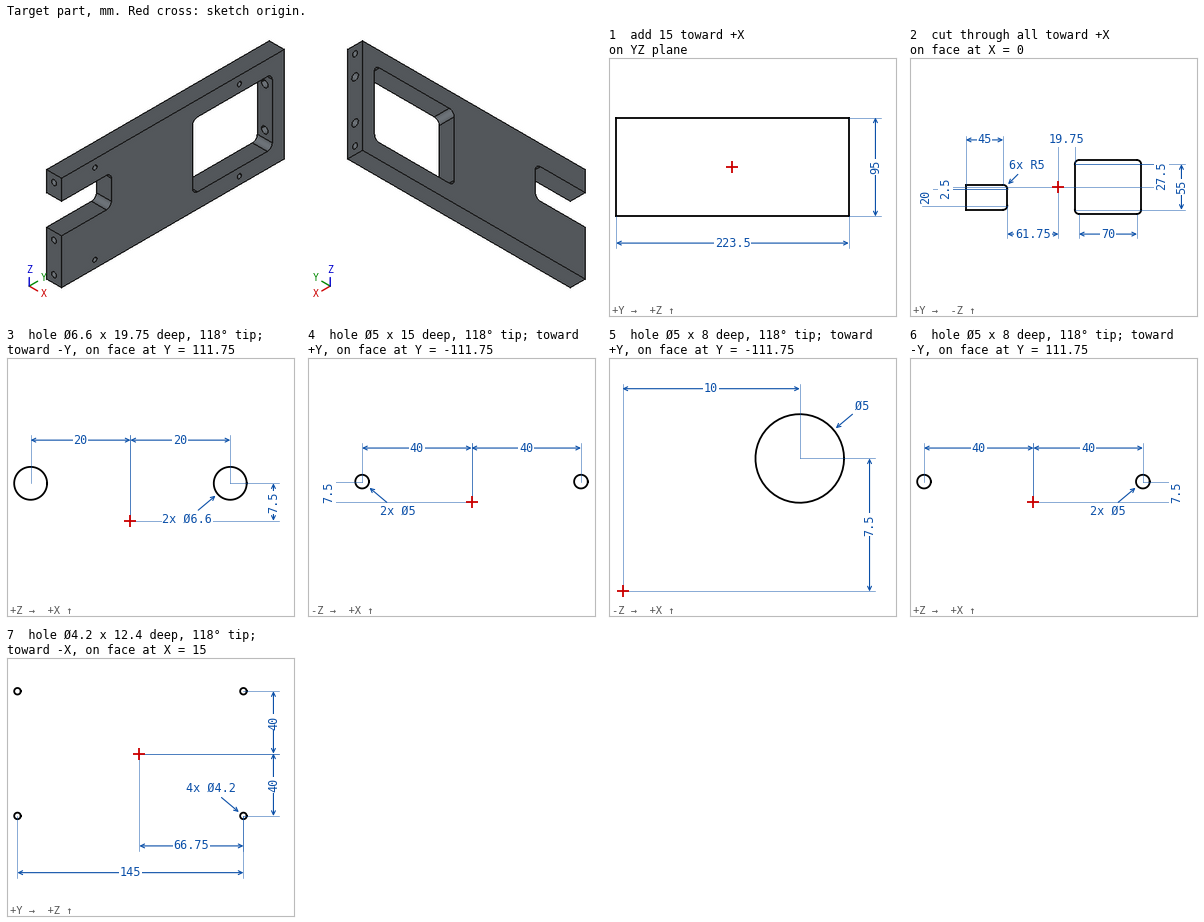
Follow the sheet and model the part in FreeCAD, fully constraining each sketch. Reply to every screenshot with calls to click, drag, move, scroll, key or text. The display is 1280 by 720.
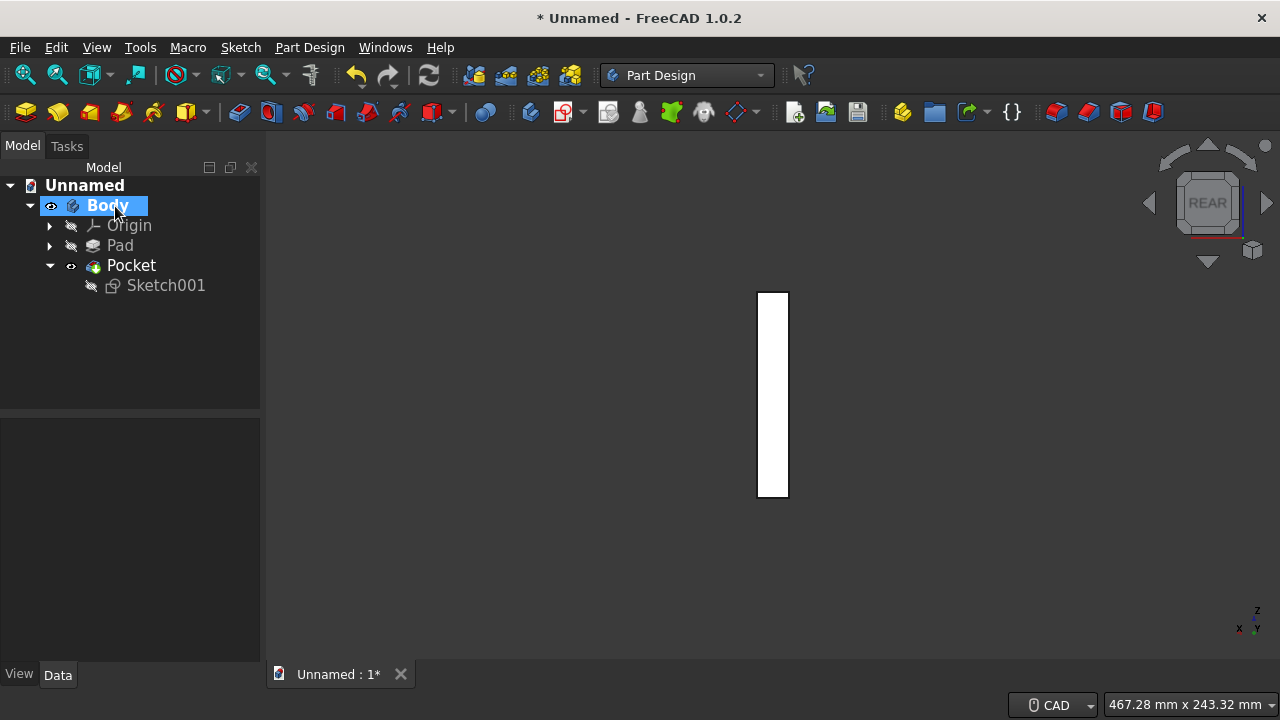
click(26, 76)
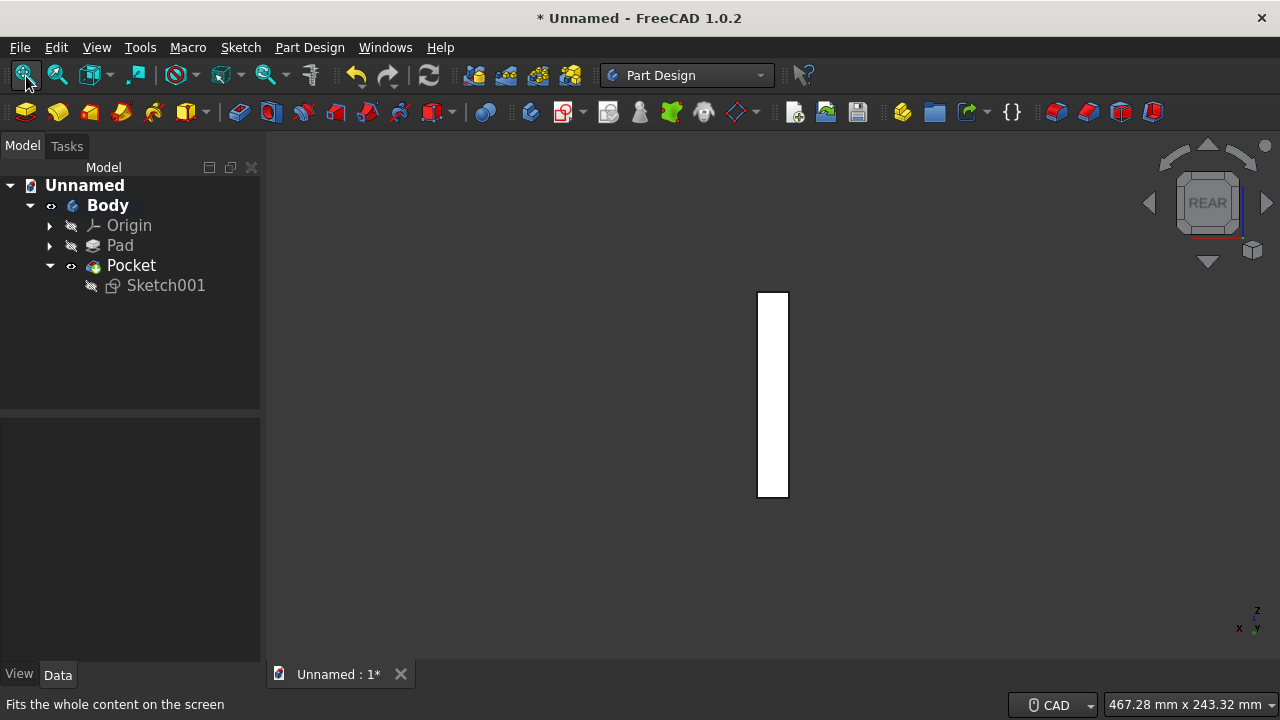
click(773, 394)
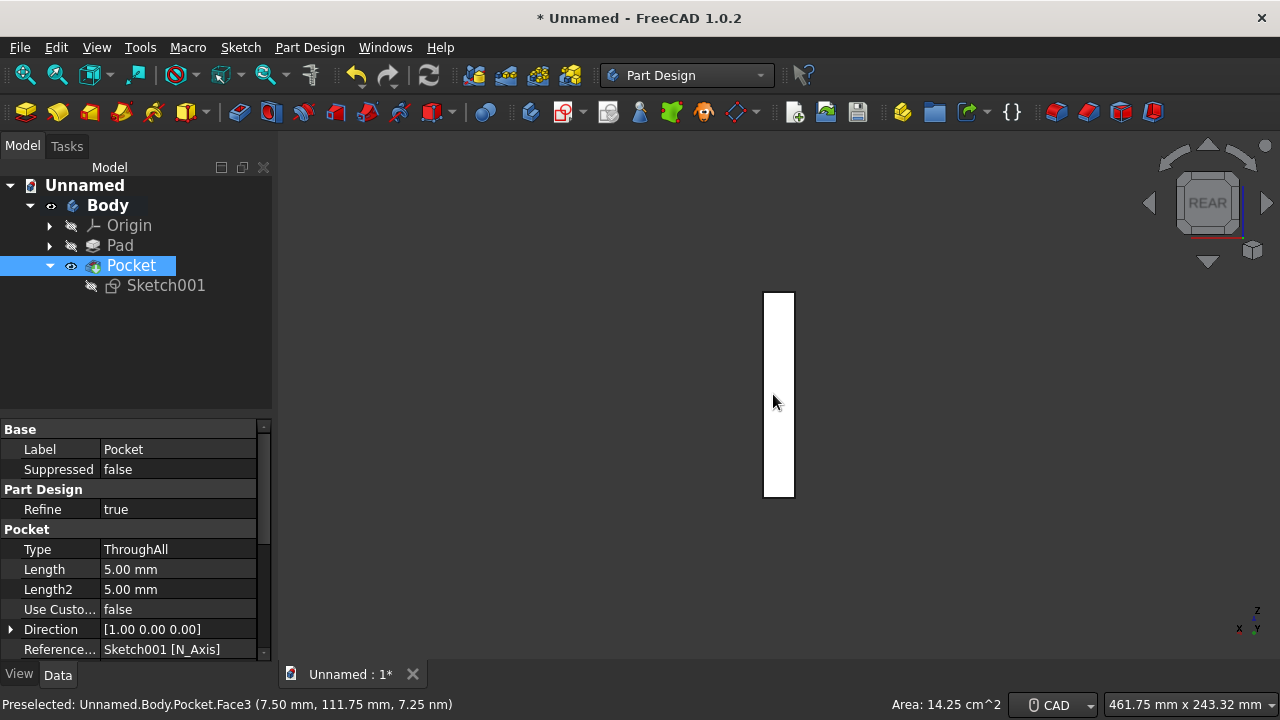
click(564, 112)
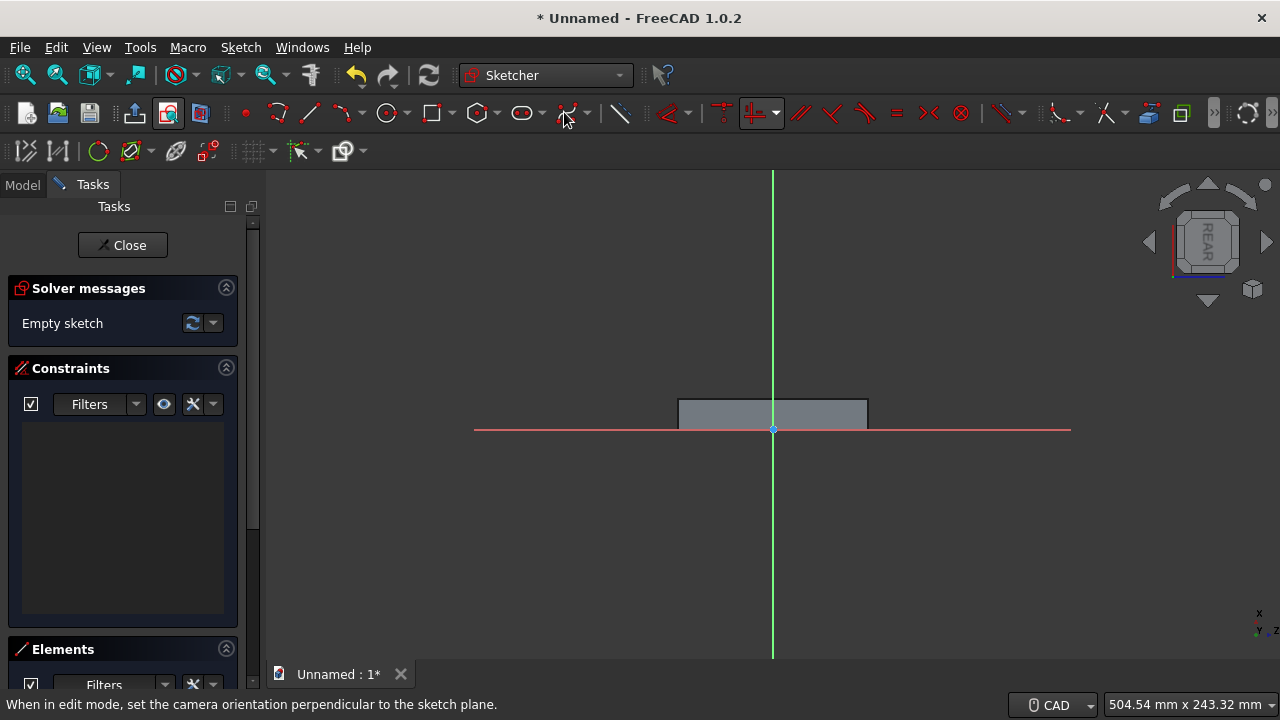
scroll(787, 420, up, 9)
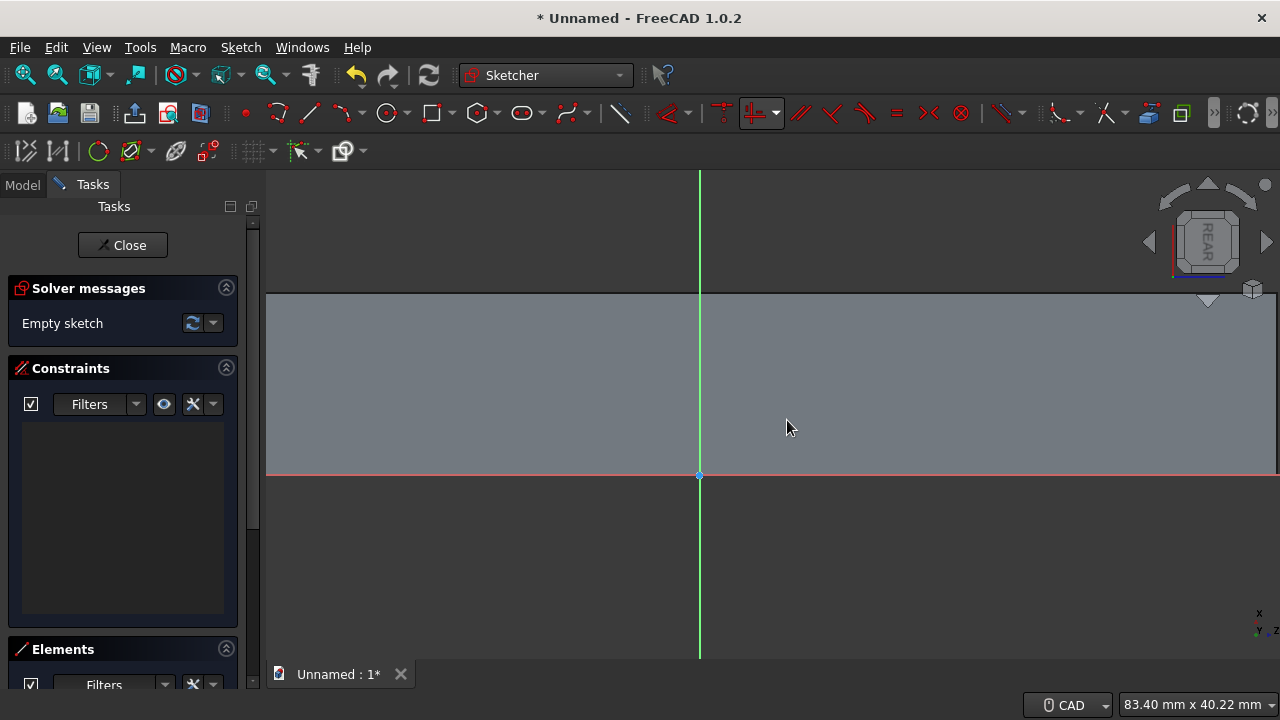
click(388, 114)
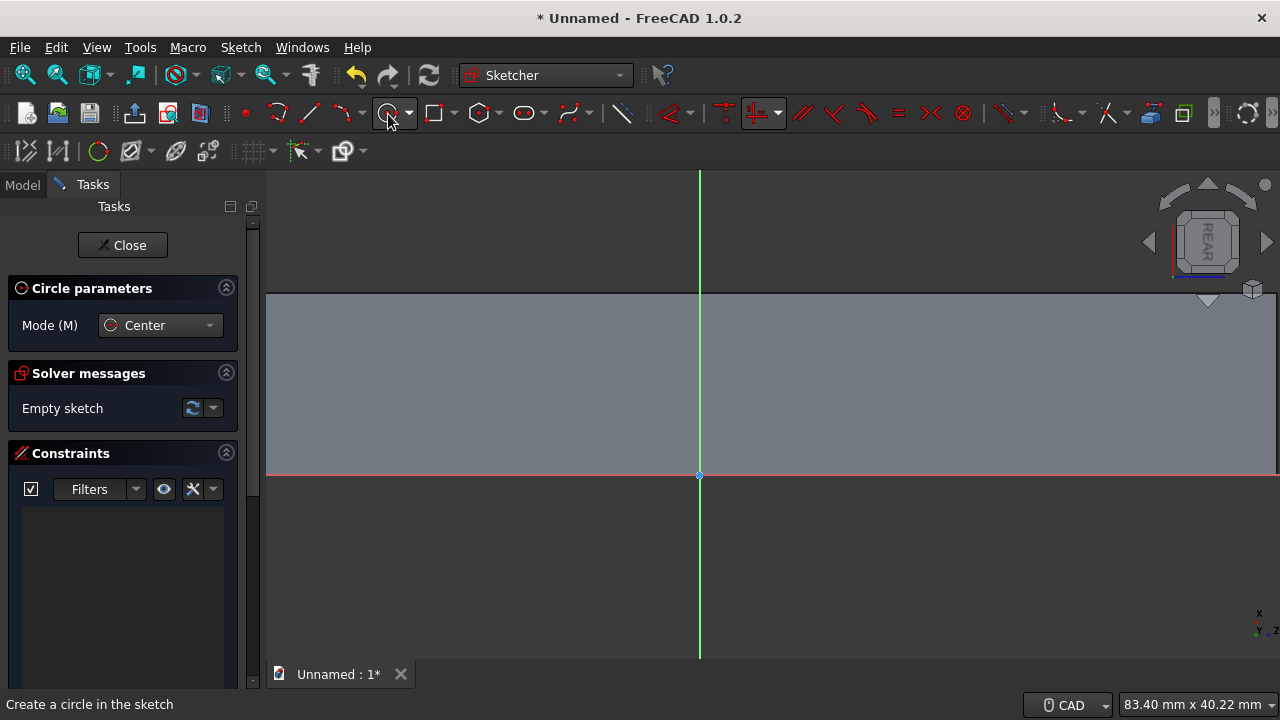
click(943, 384)
move(971, 356)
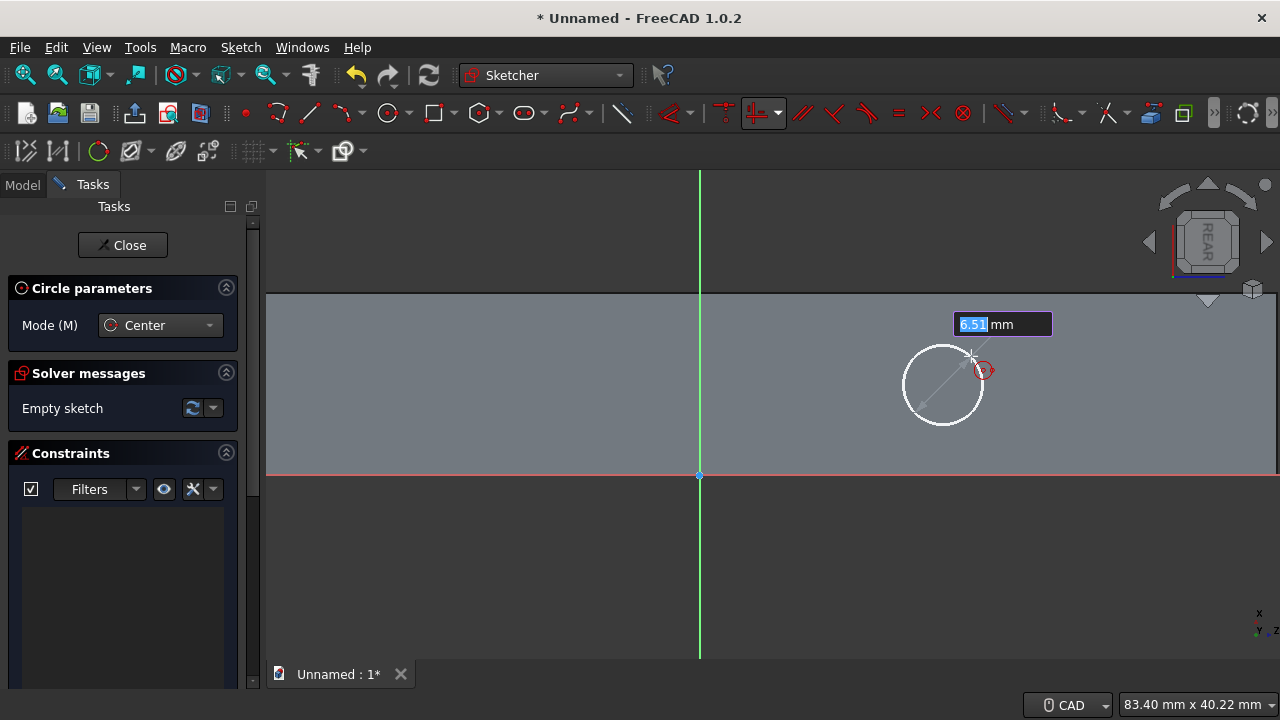
text(6.6)
key(Return)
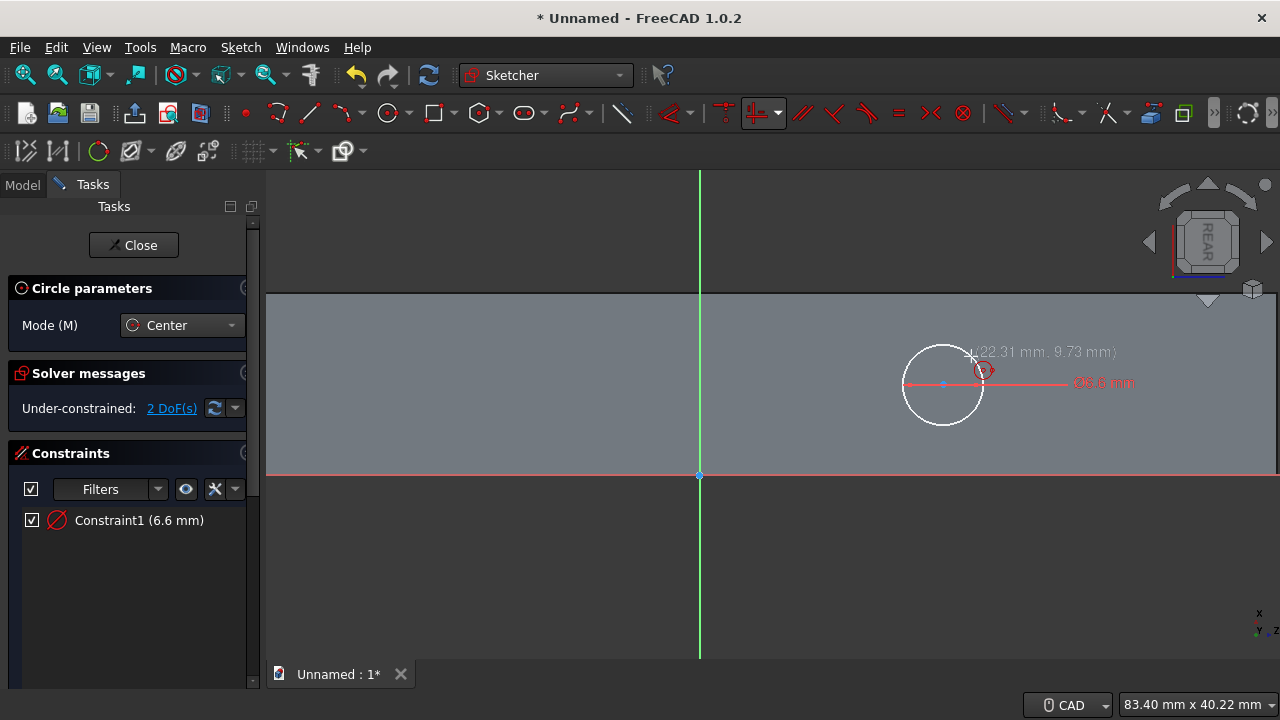
click(457, 384)
move(485, 356)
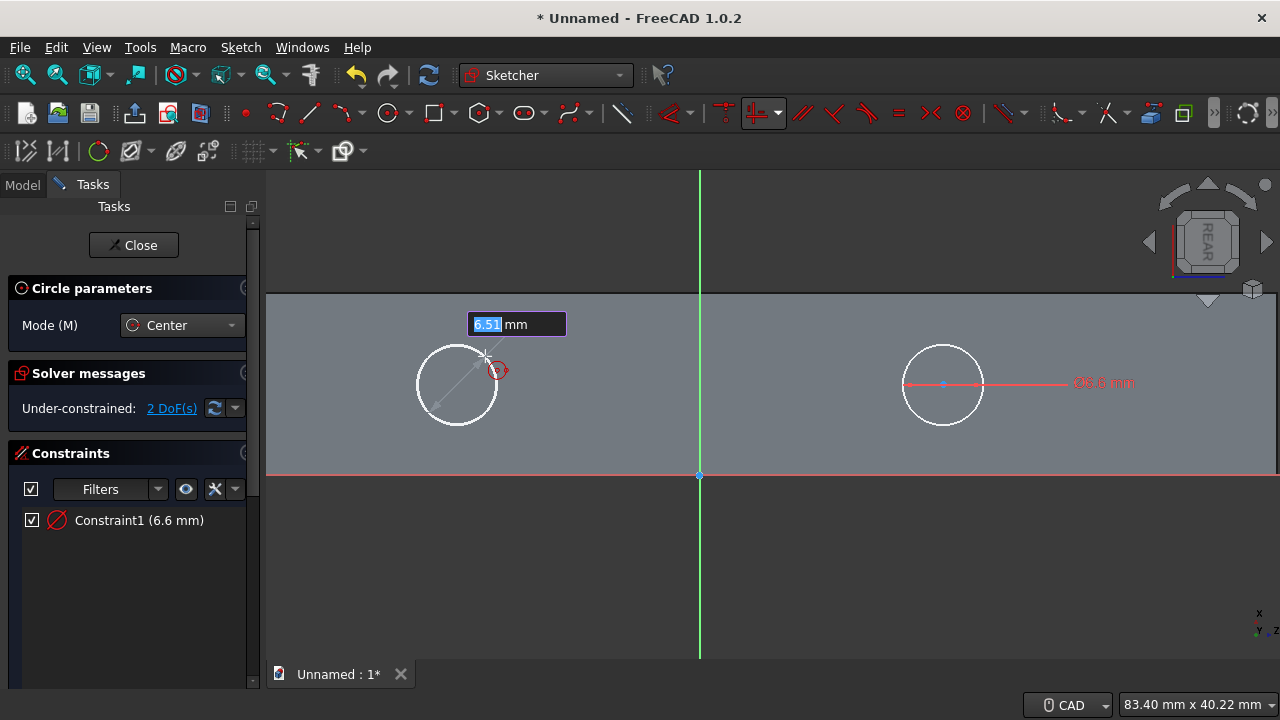
text(6.6)
key(Return)
key(Escape)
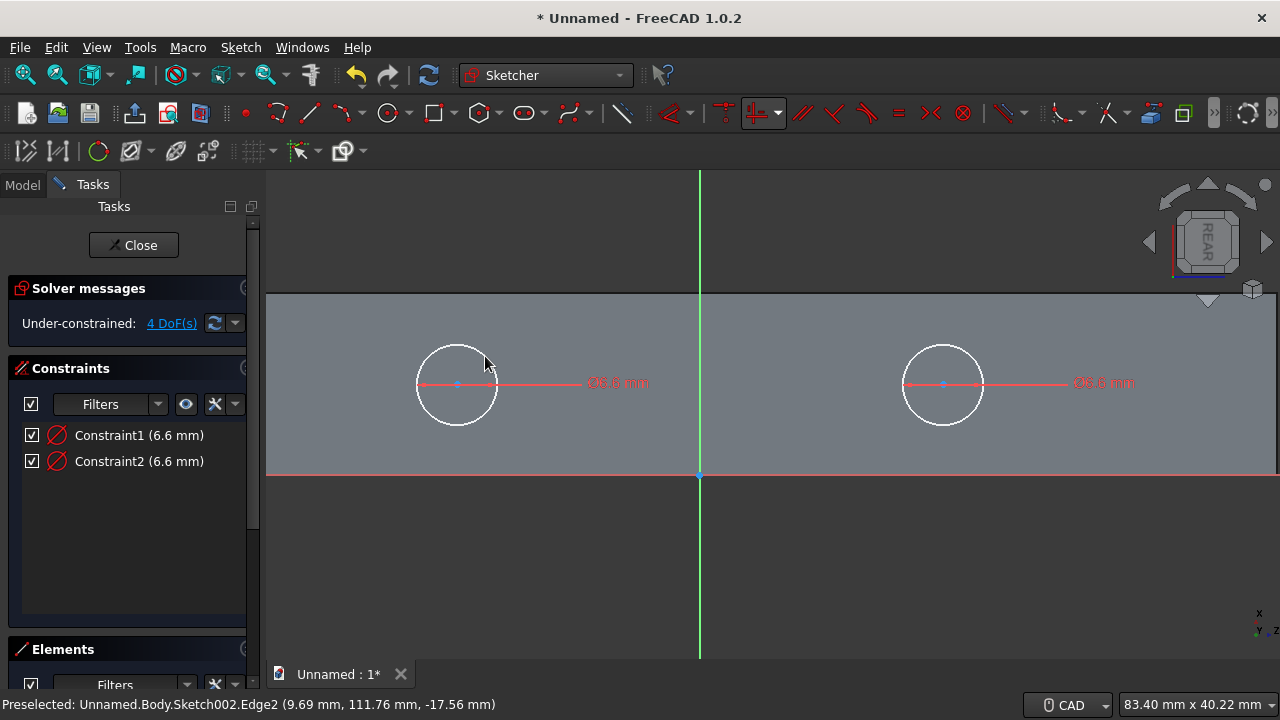
click(943, 385)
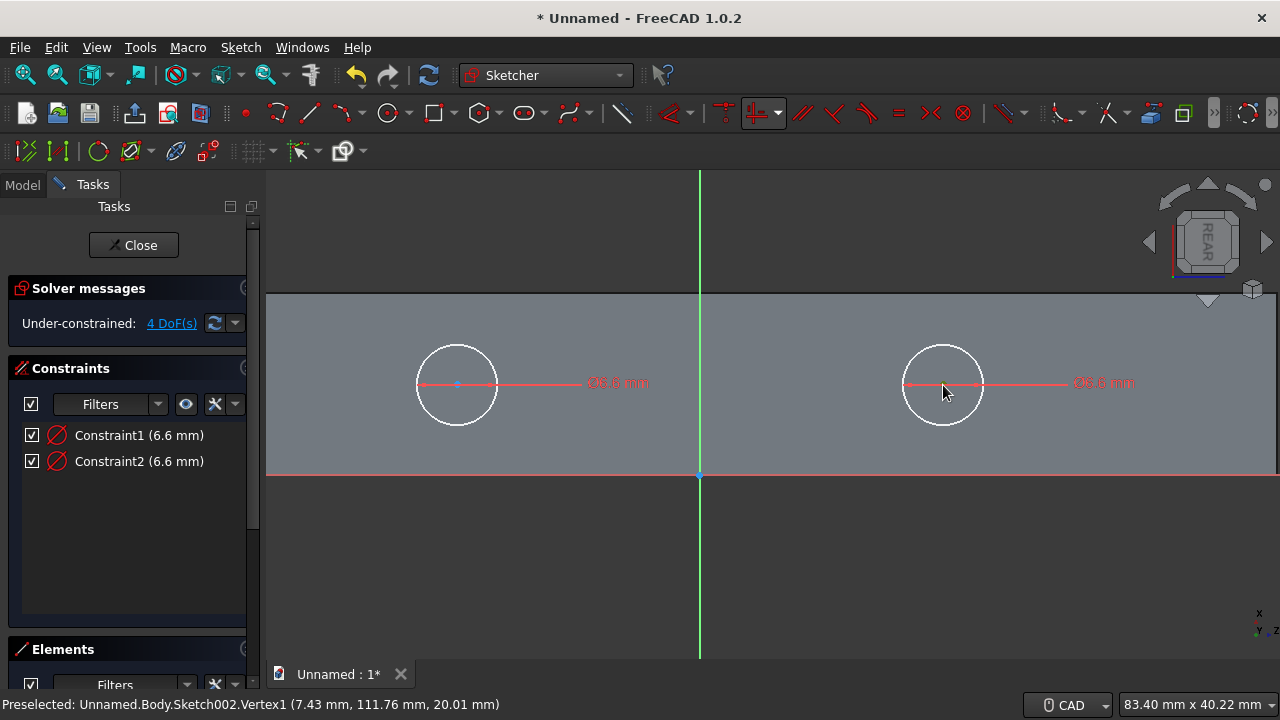
click(457, 385)